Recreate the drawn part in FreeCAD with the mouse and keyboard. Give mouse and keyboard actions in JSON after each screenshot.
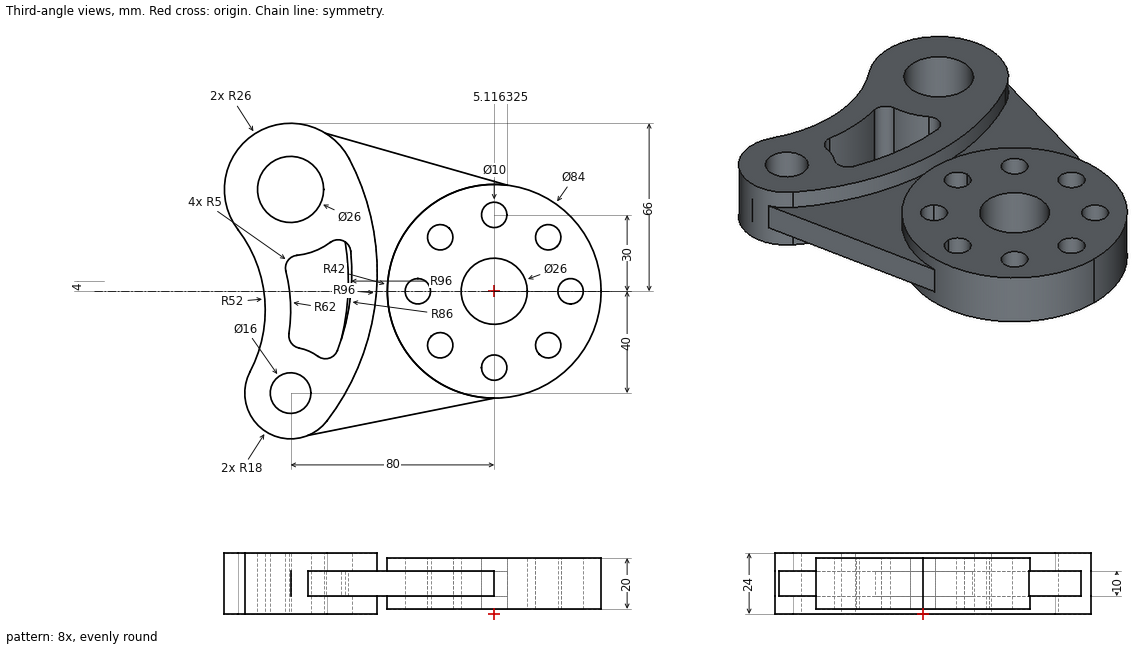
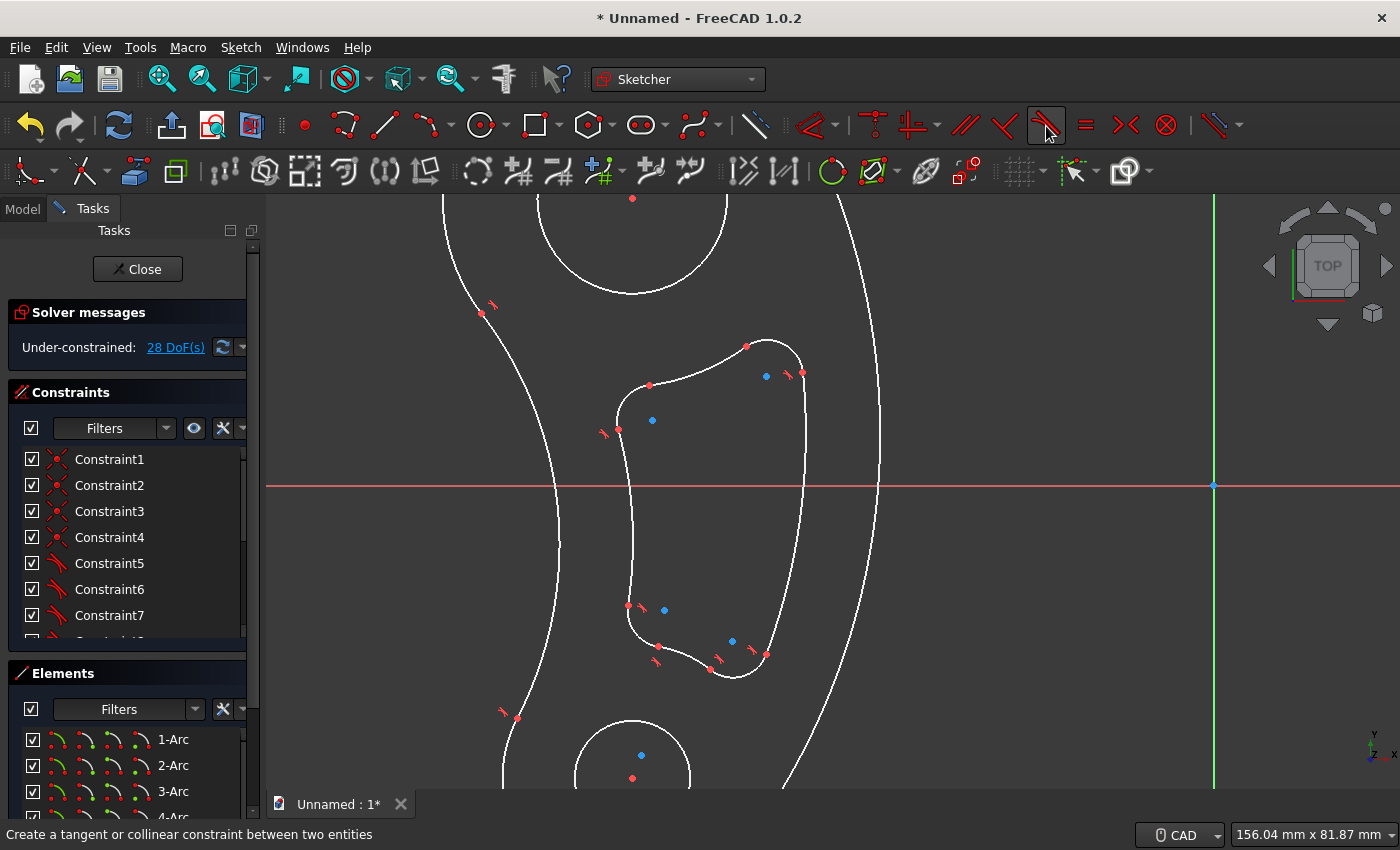
{"action": "left_click", "coordinate": [632, 392]}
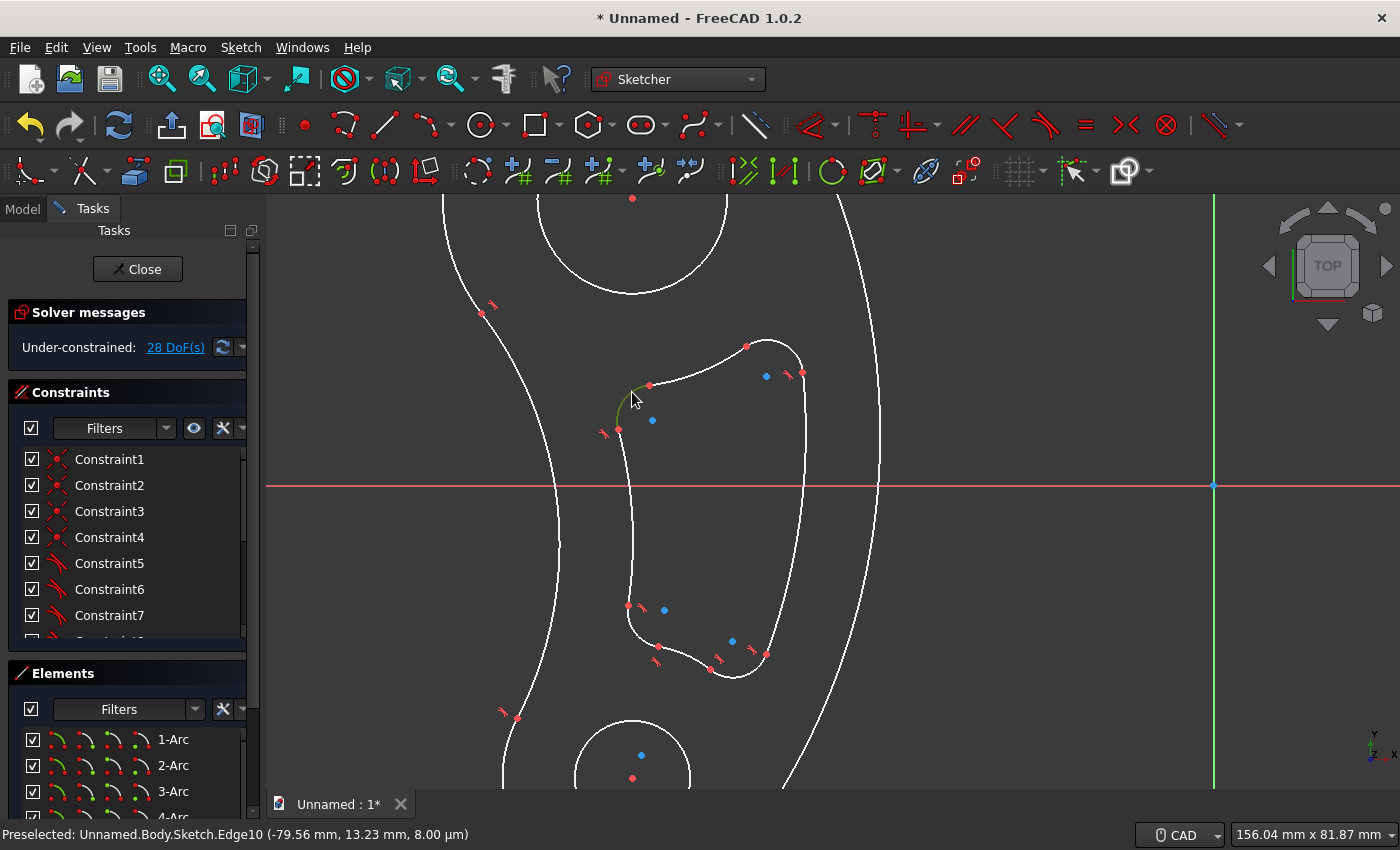
{"action": "left_click", "coordinate": [680, 379]}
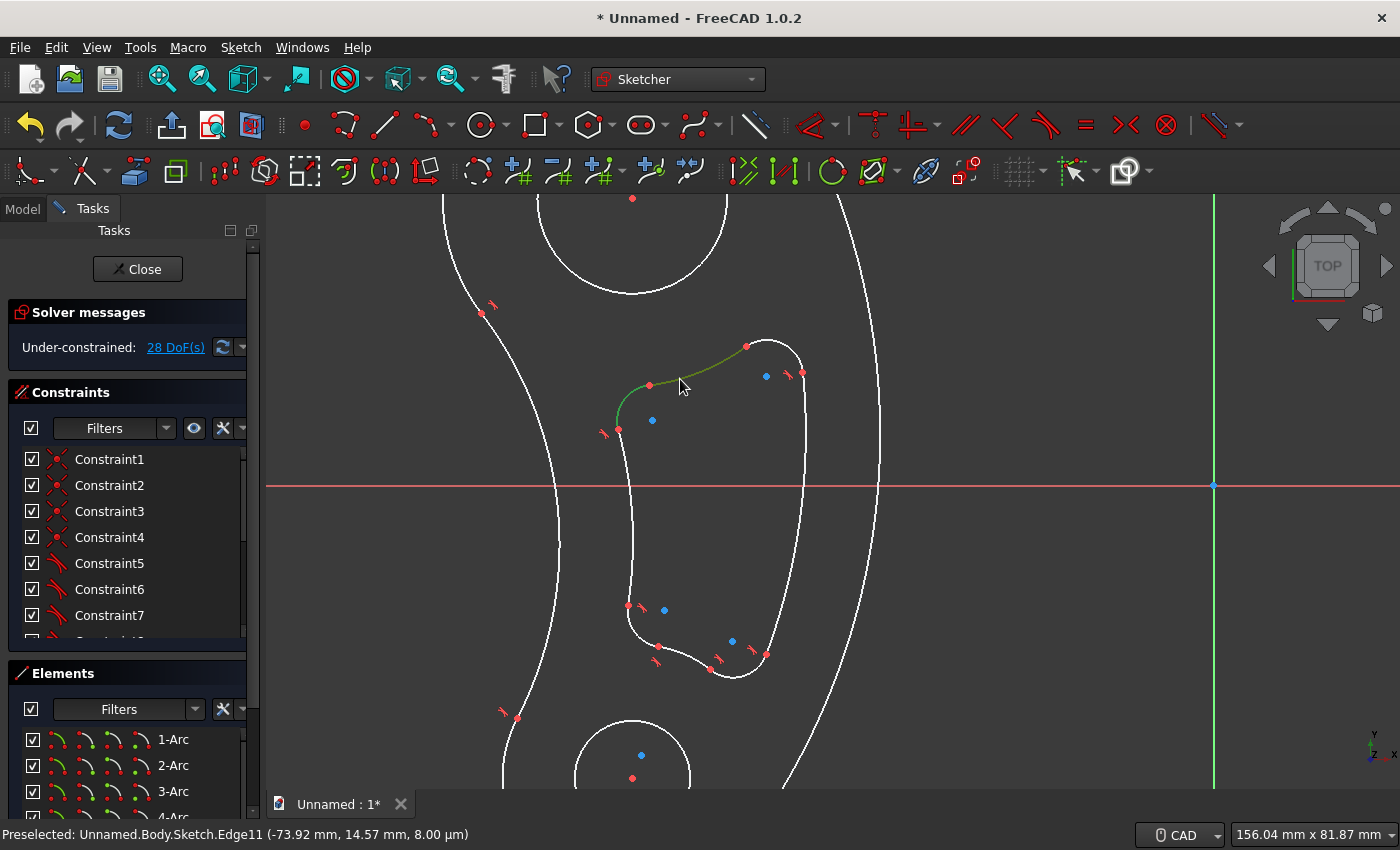
{"action": "left_click", "coordinate": [1046, 126]}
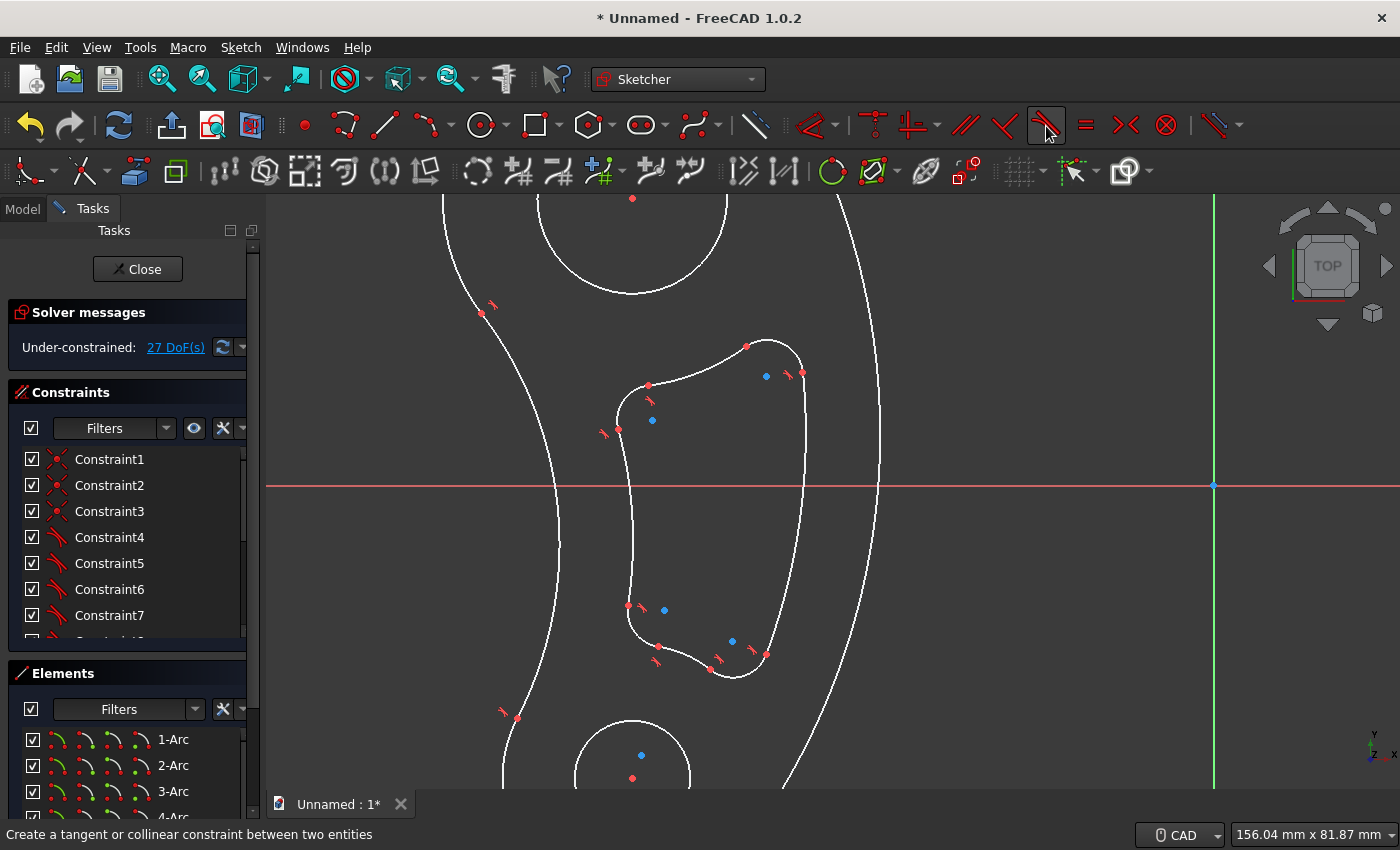
{"action": "left_click", "coordinate": [679, 379]}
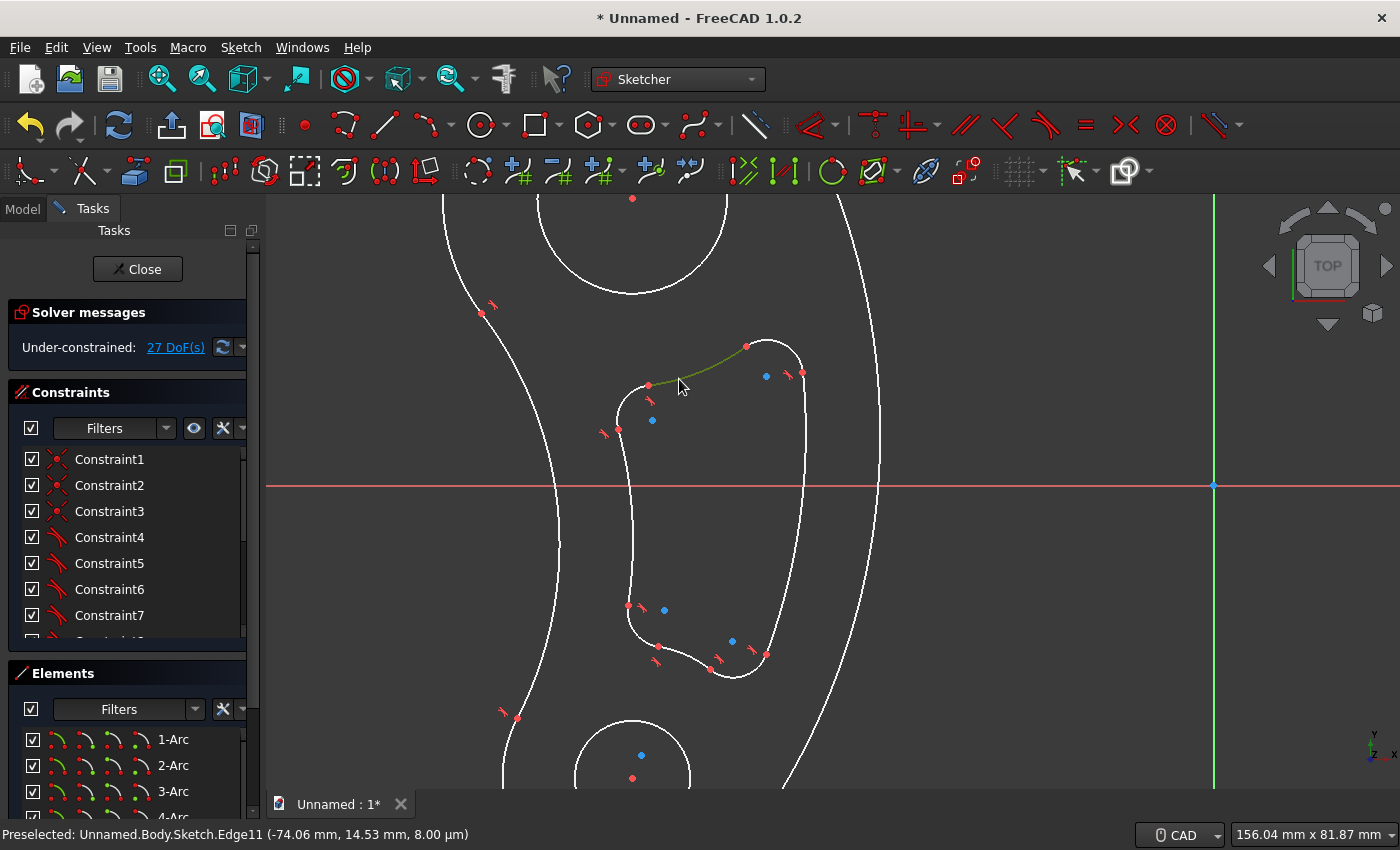
{"action": "left_click", "coordinate": [794, 352]}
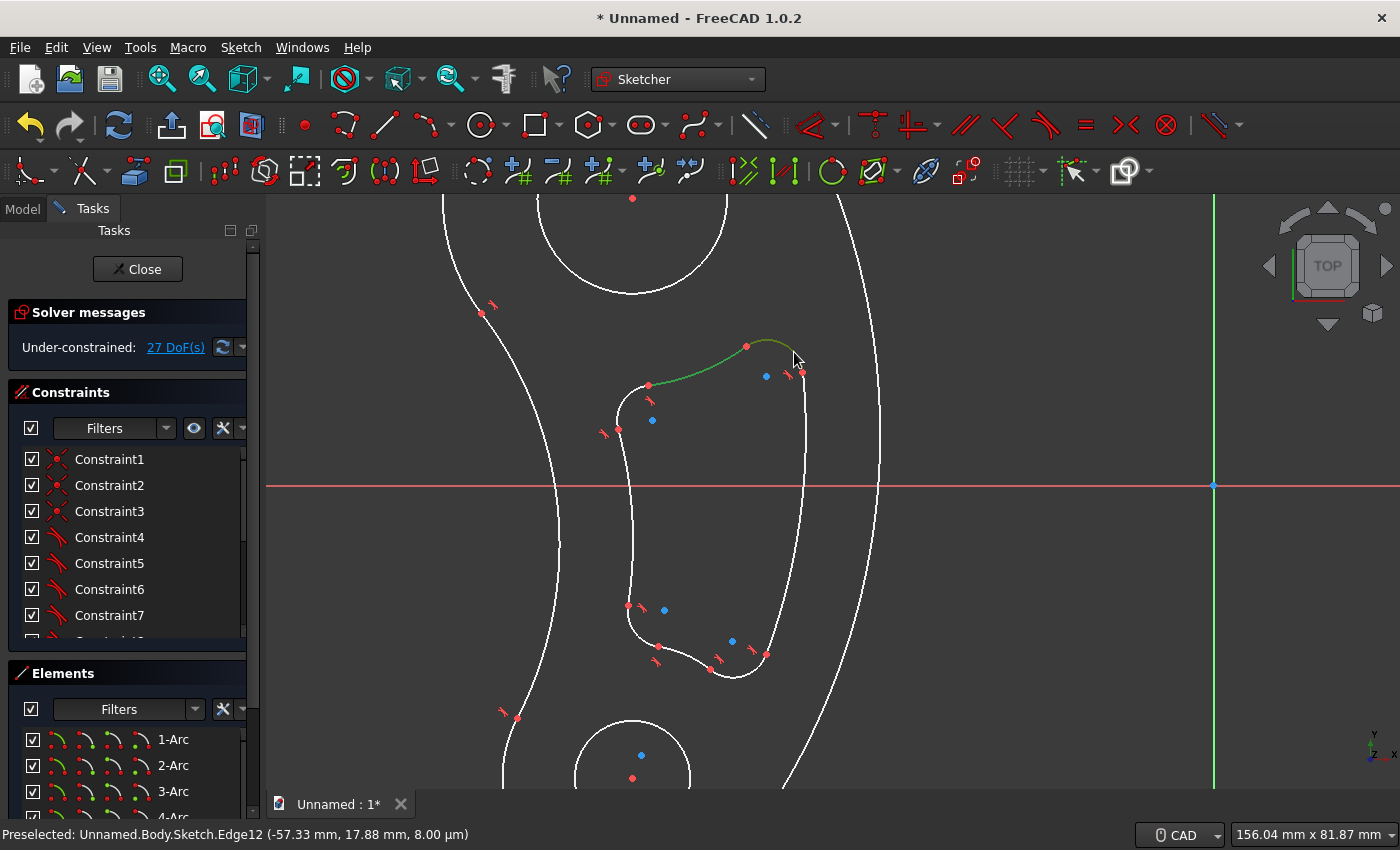
{"action": "left_click", "coordinate": [1046, 126]}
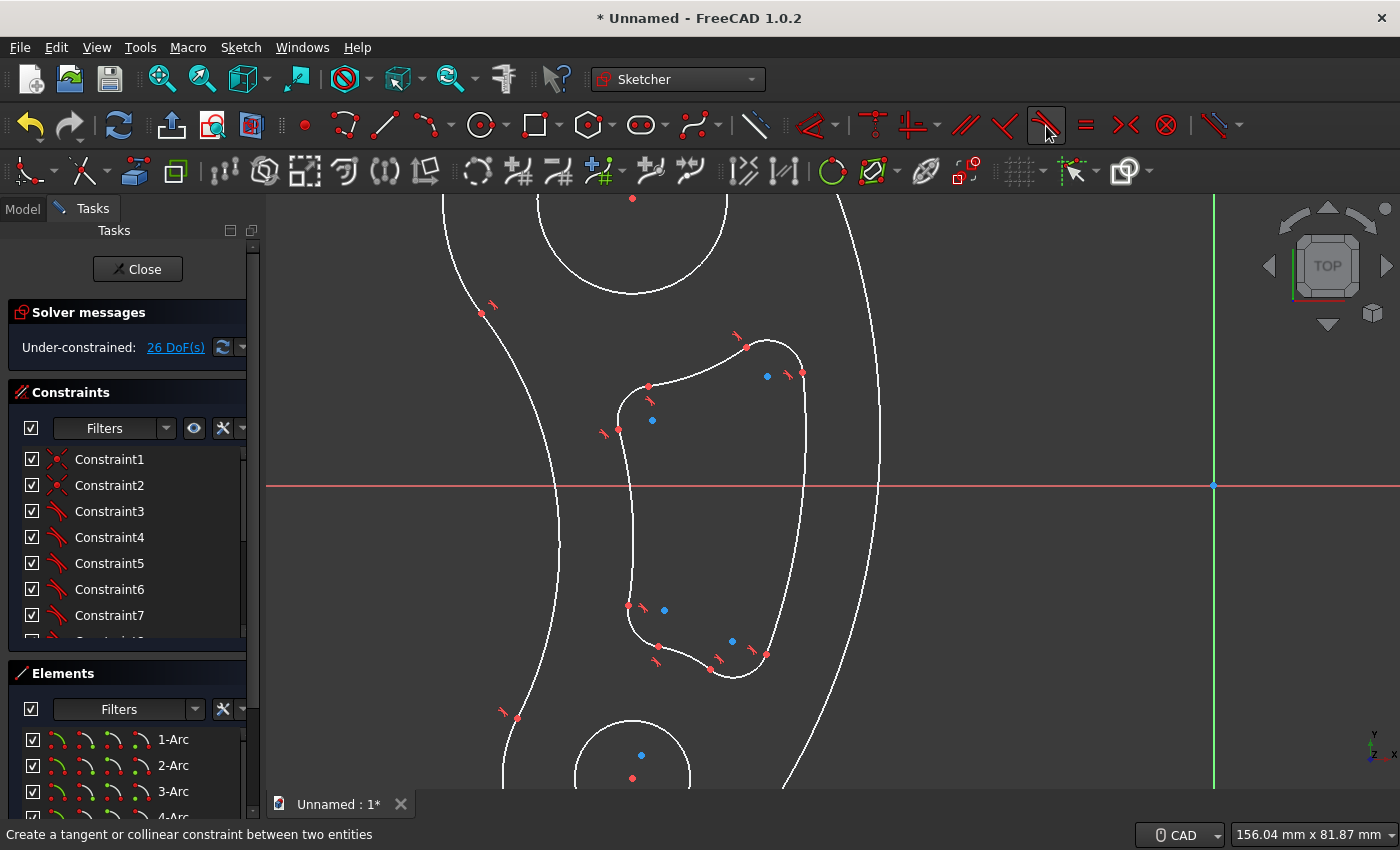
{"action": "left_click", "coordinate": [846, 649]}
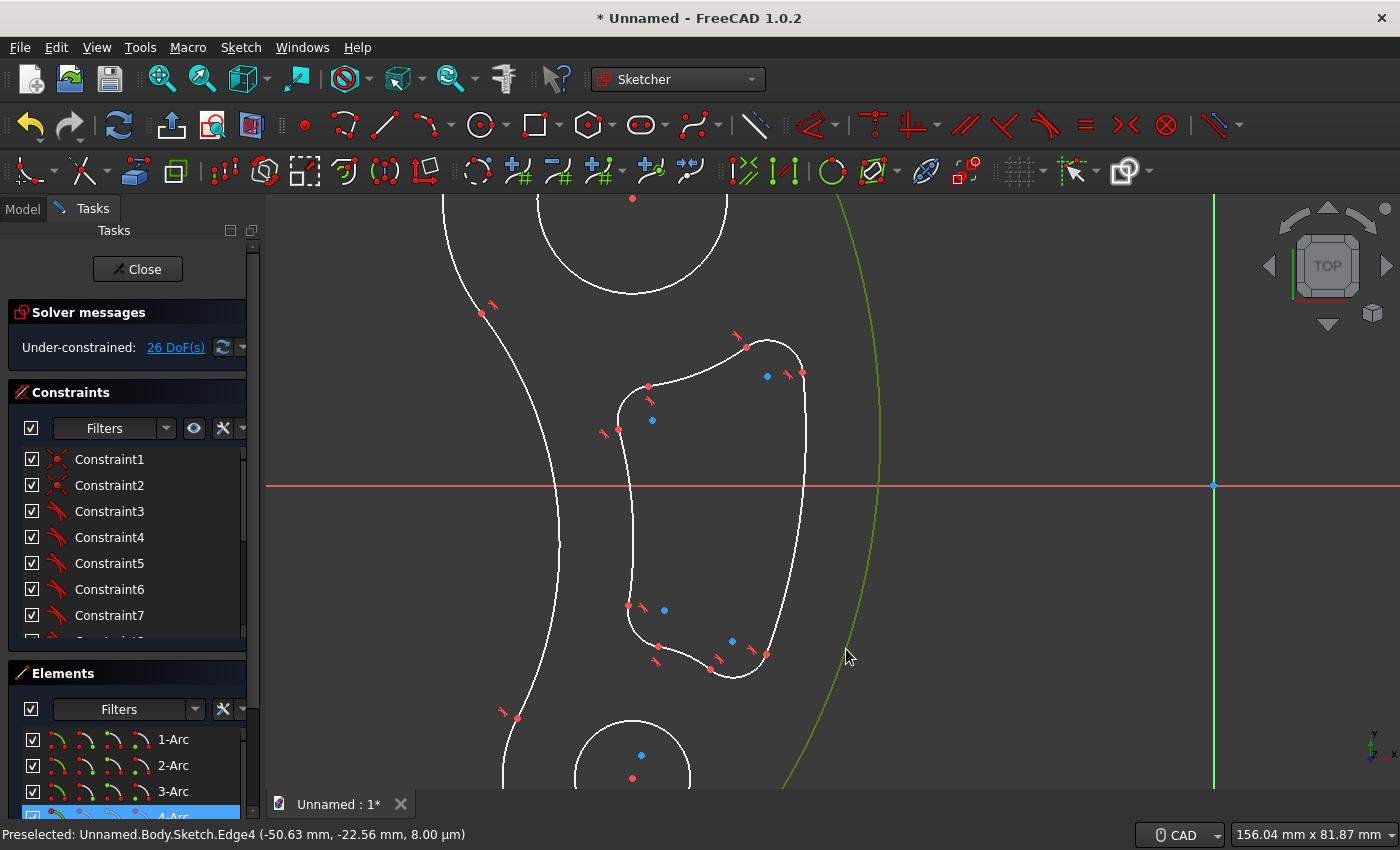
{"action": "left_click", "coordinate": [791, 572]}